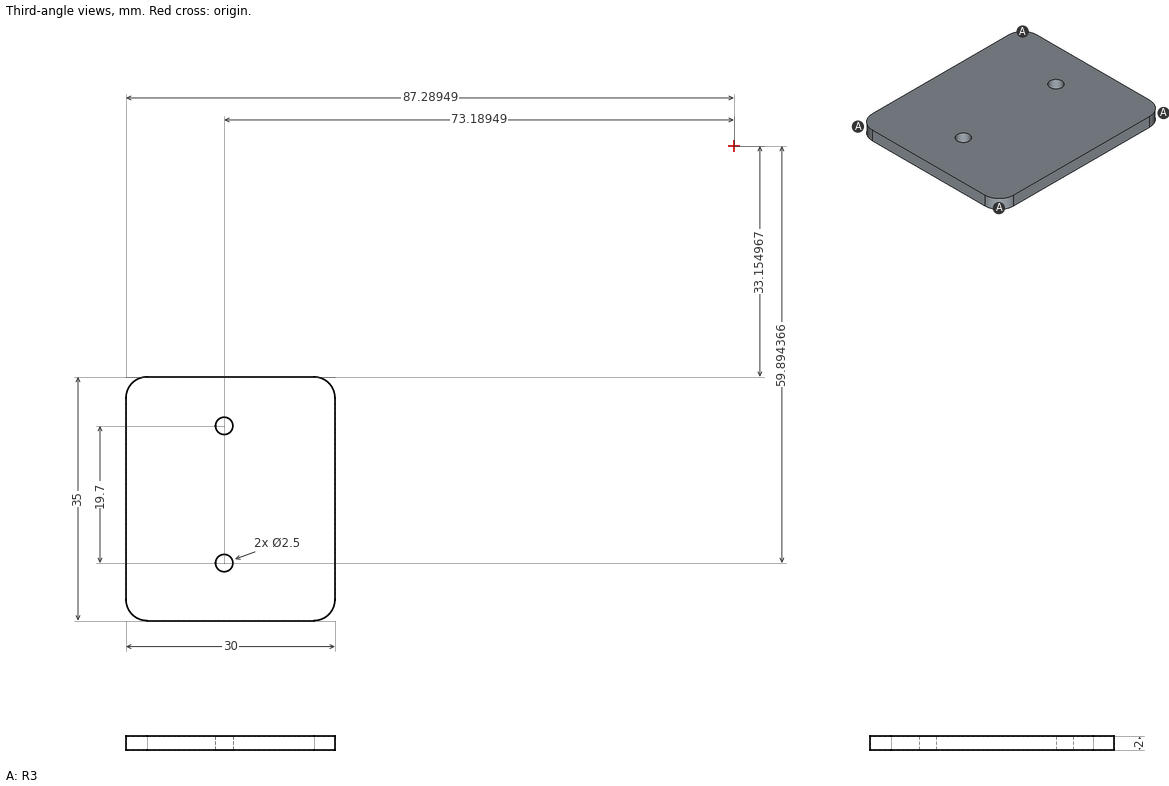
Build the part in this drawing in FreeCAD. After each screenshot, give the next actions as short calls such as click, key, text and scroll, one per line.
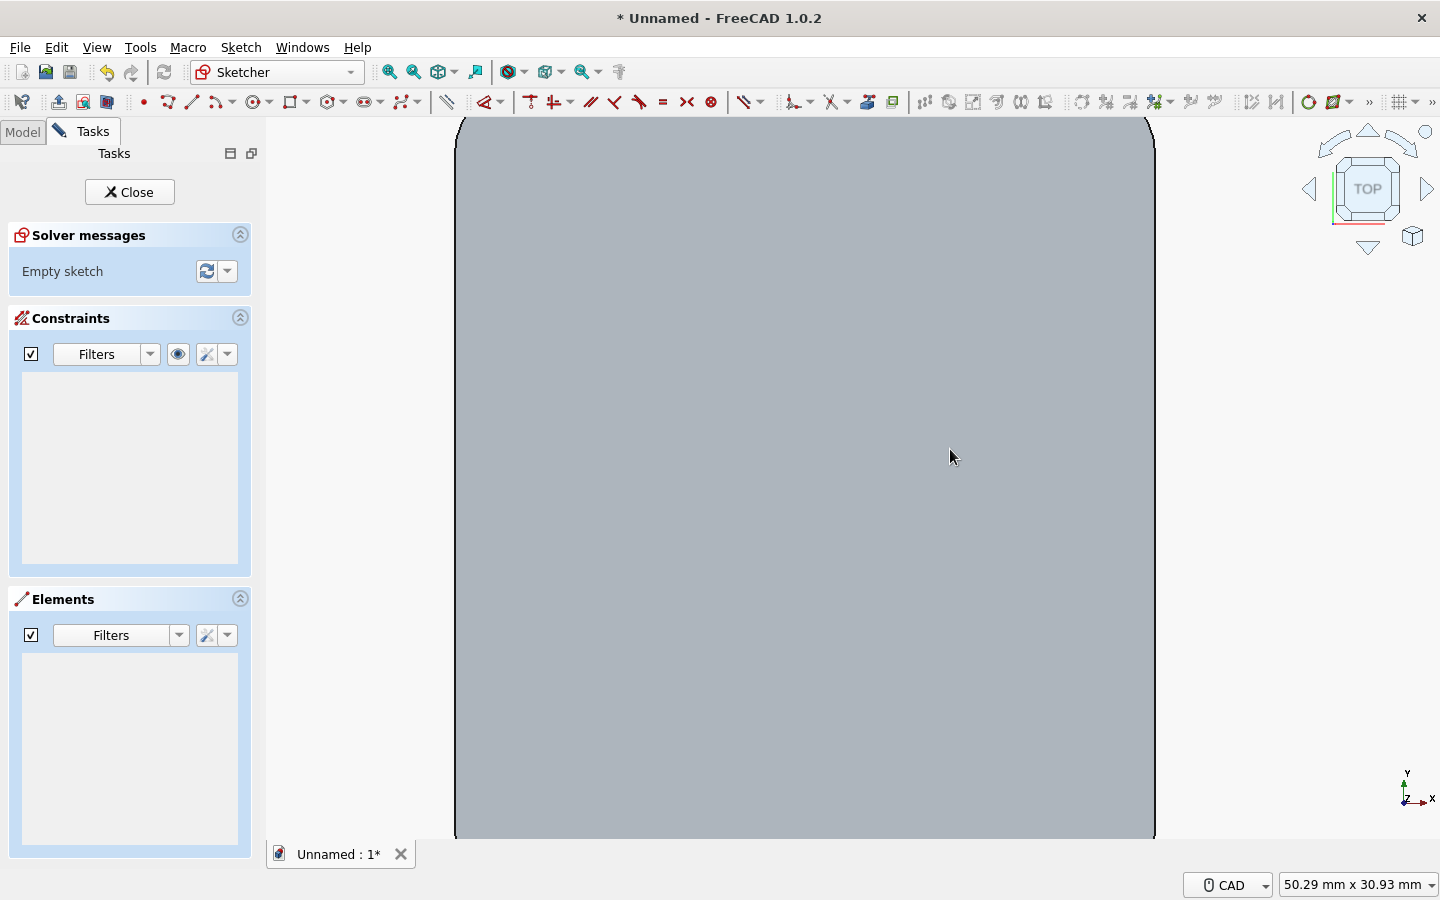
click(254, 102)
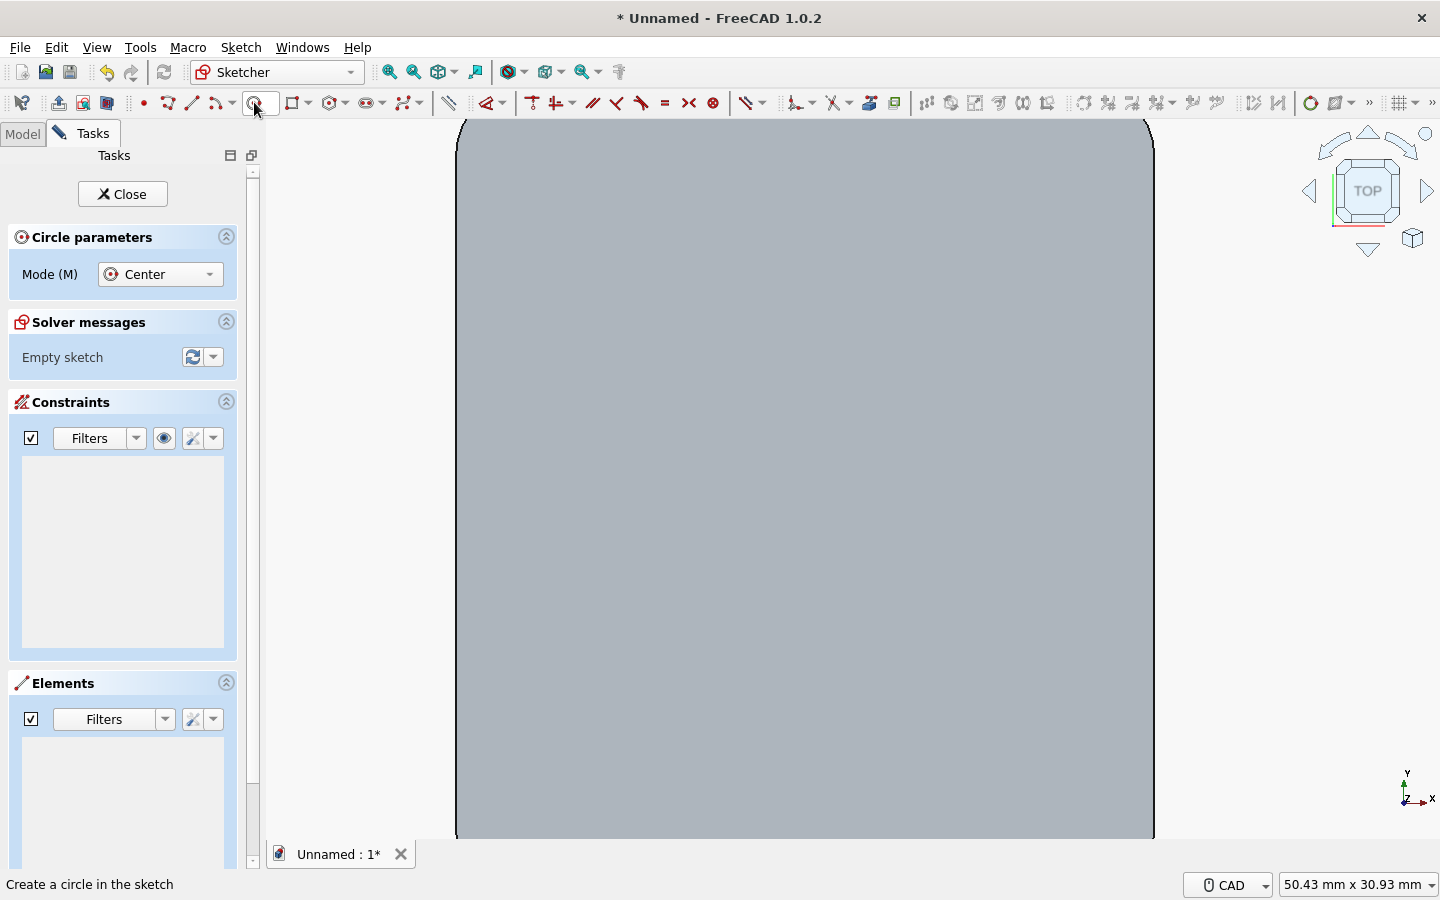
click(784, 708)
move(805, 688)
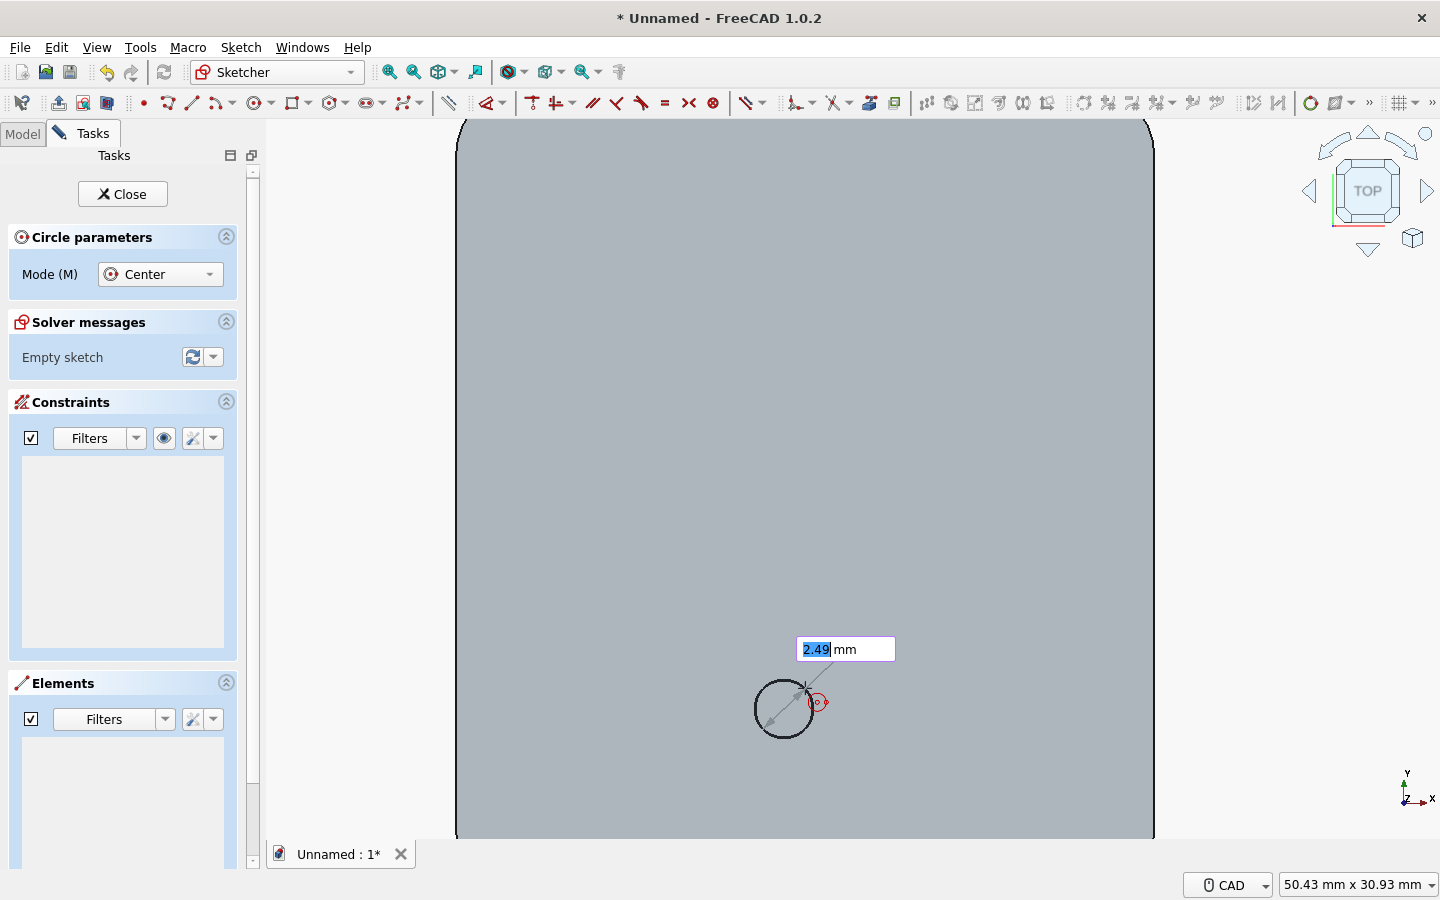
text(2.5)
key(Return)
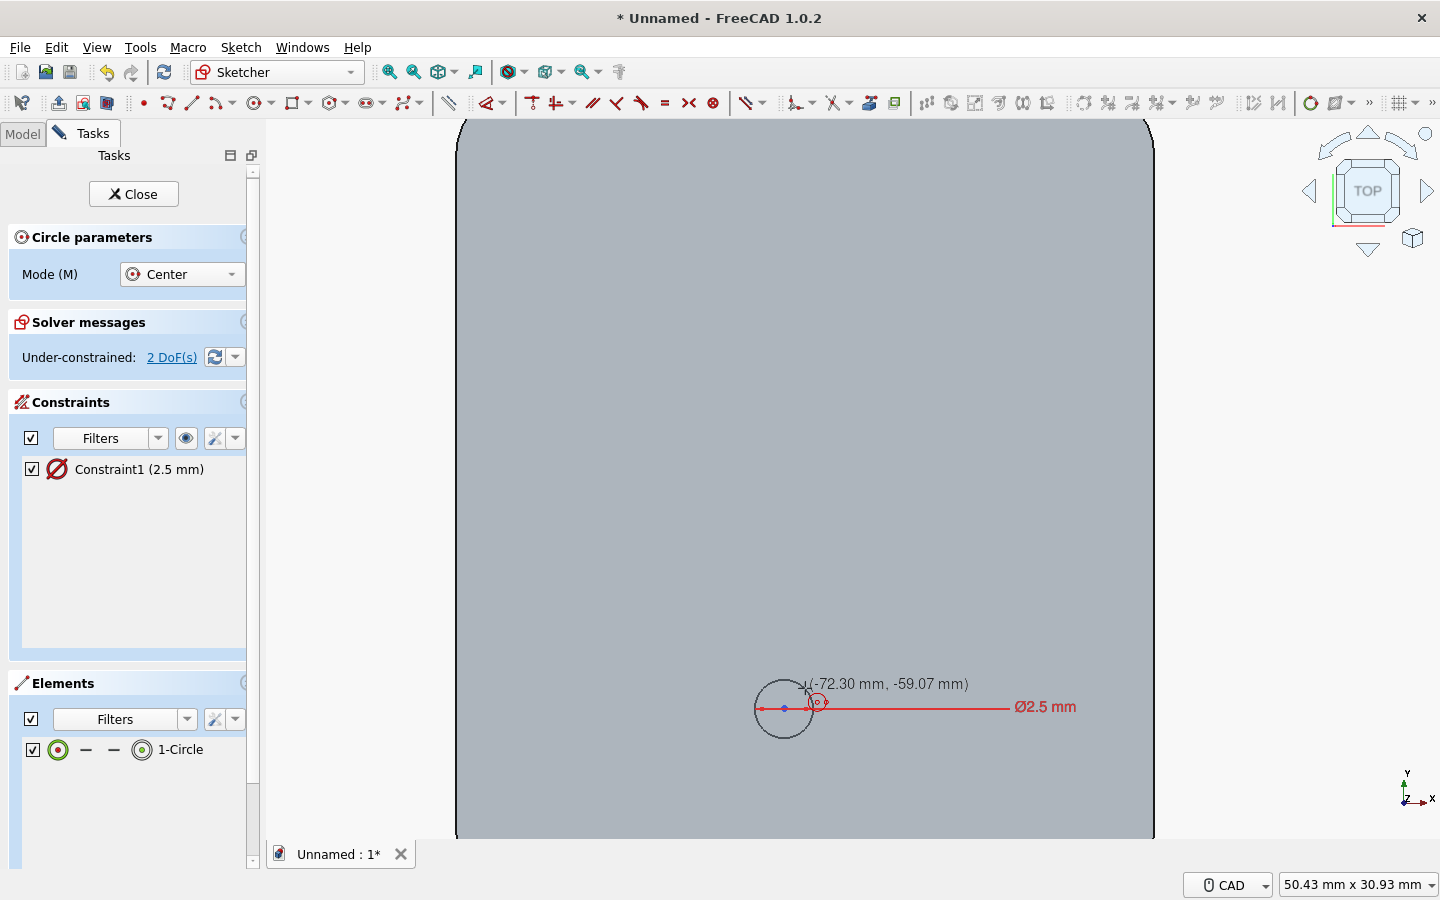
click(784, 249)
move(805, 229)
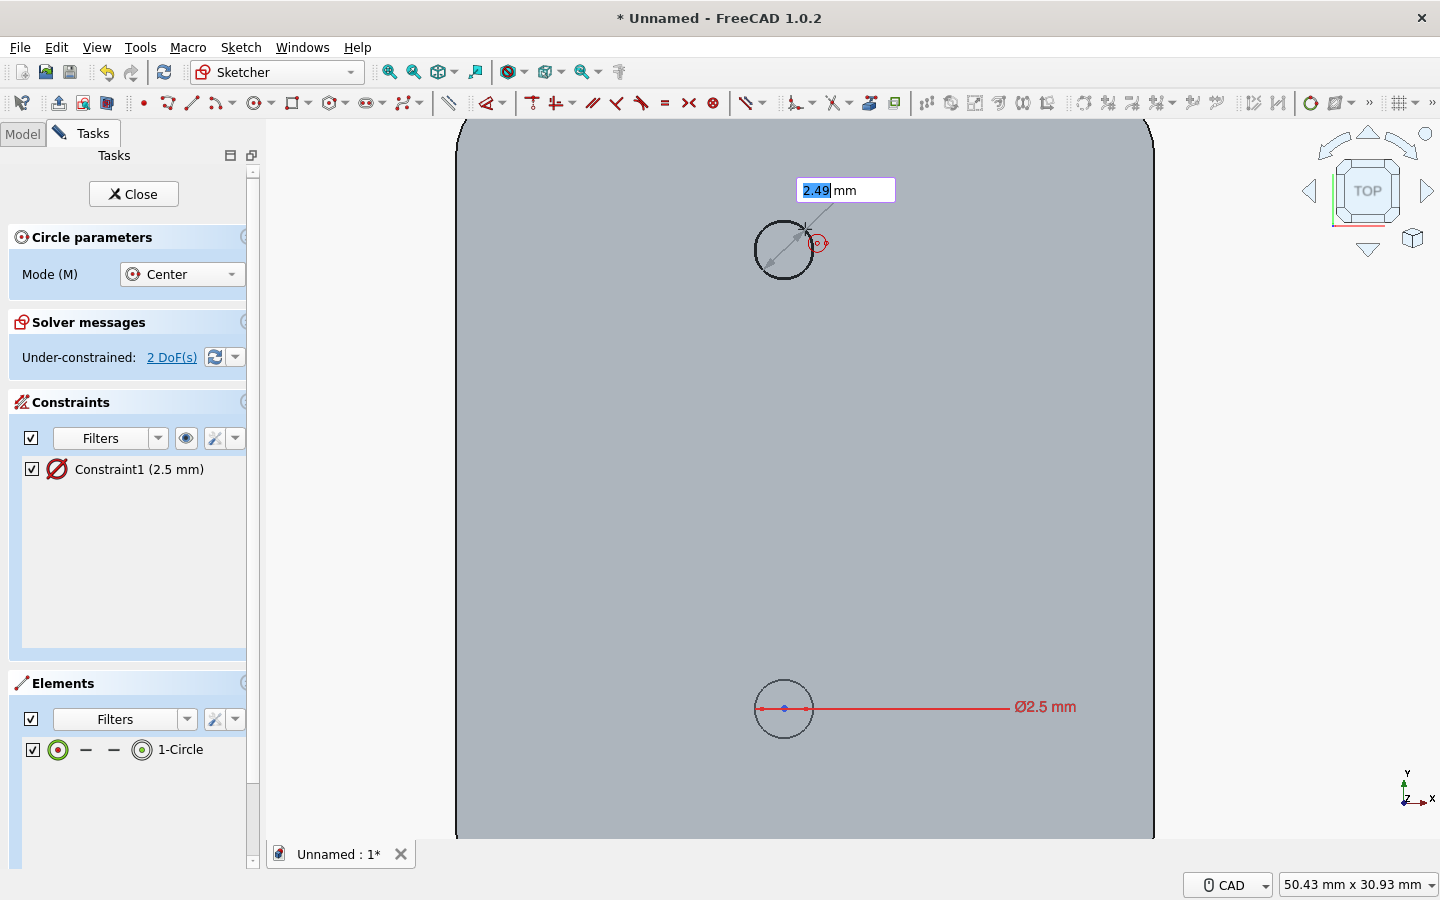
text(2.5)
key(Return)
key(Escape)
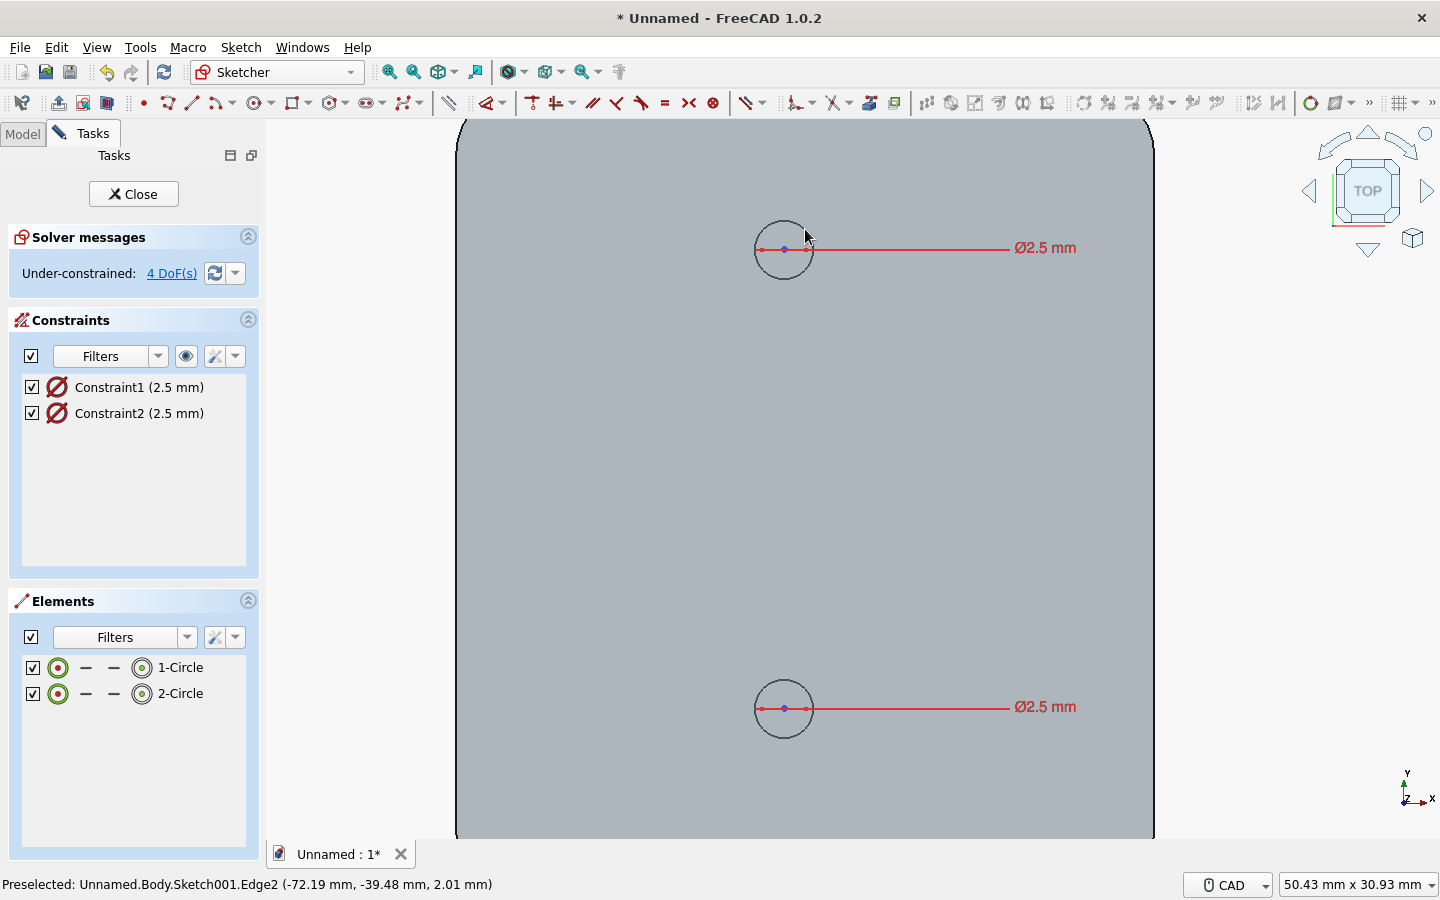
click(784, 709)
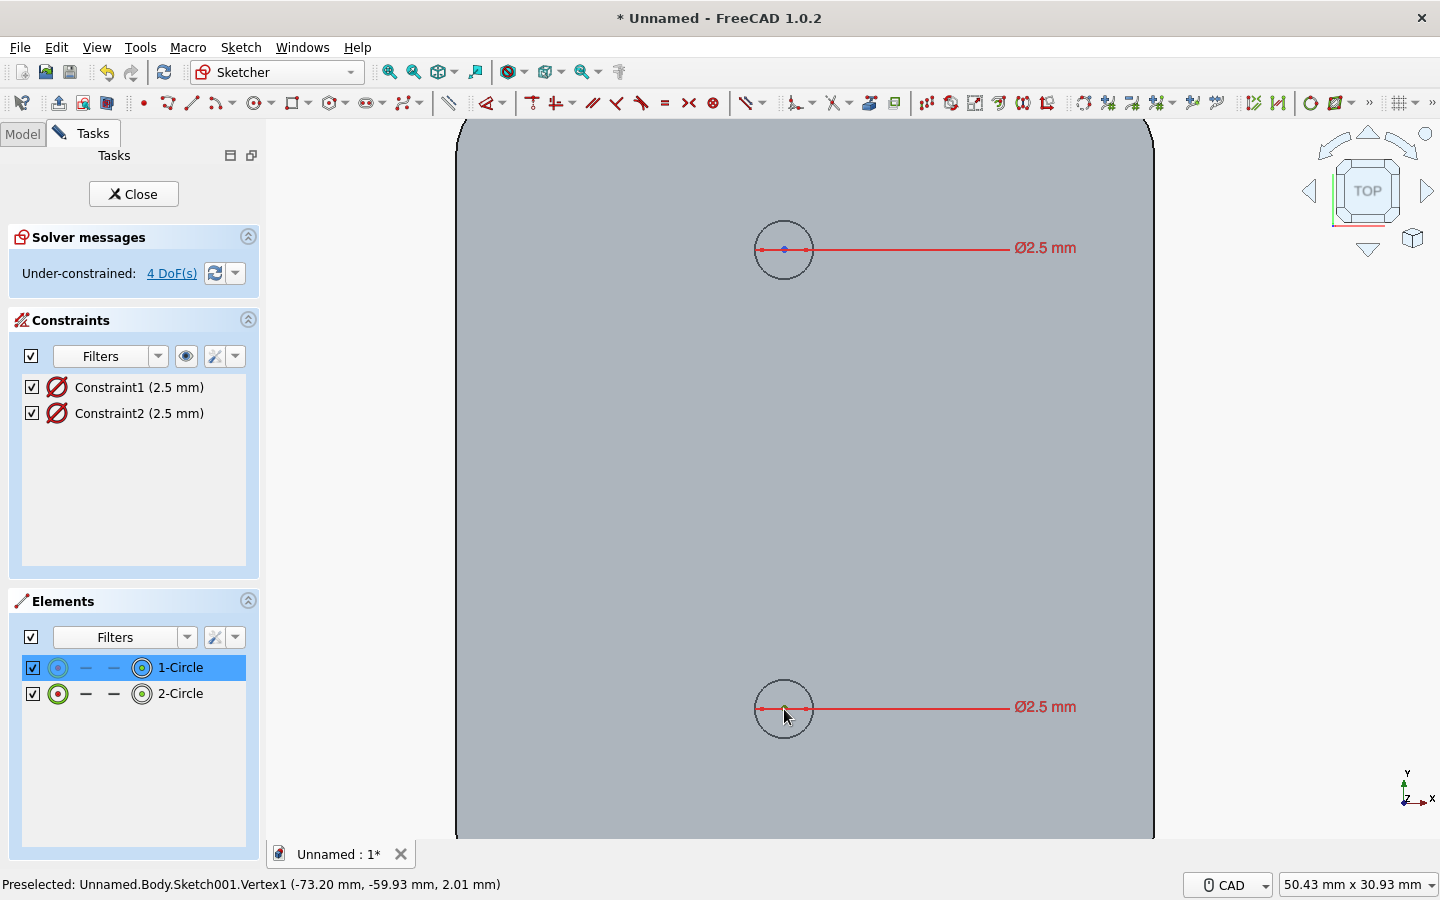
click(784, 250)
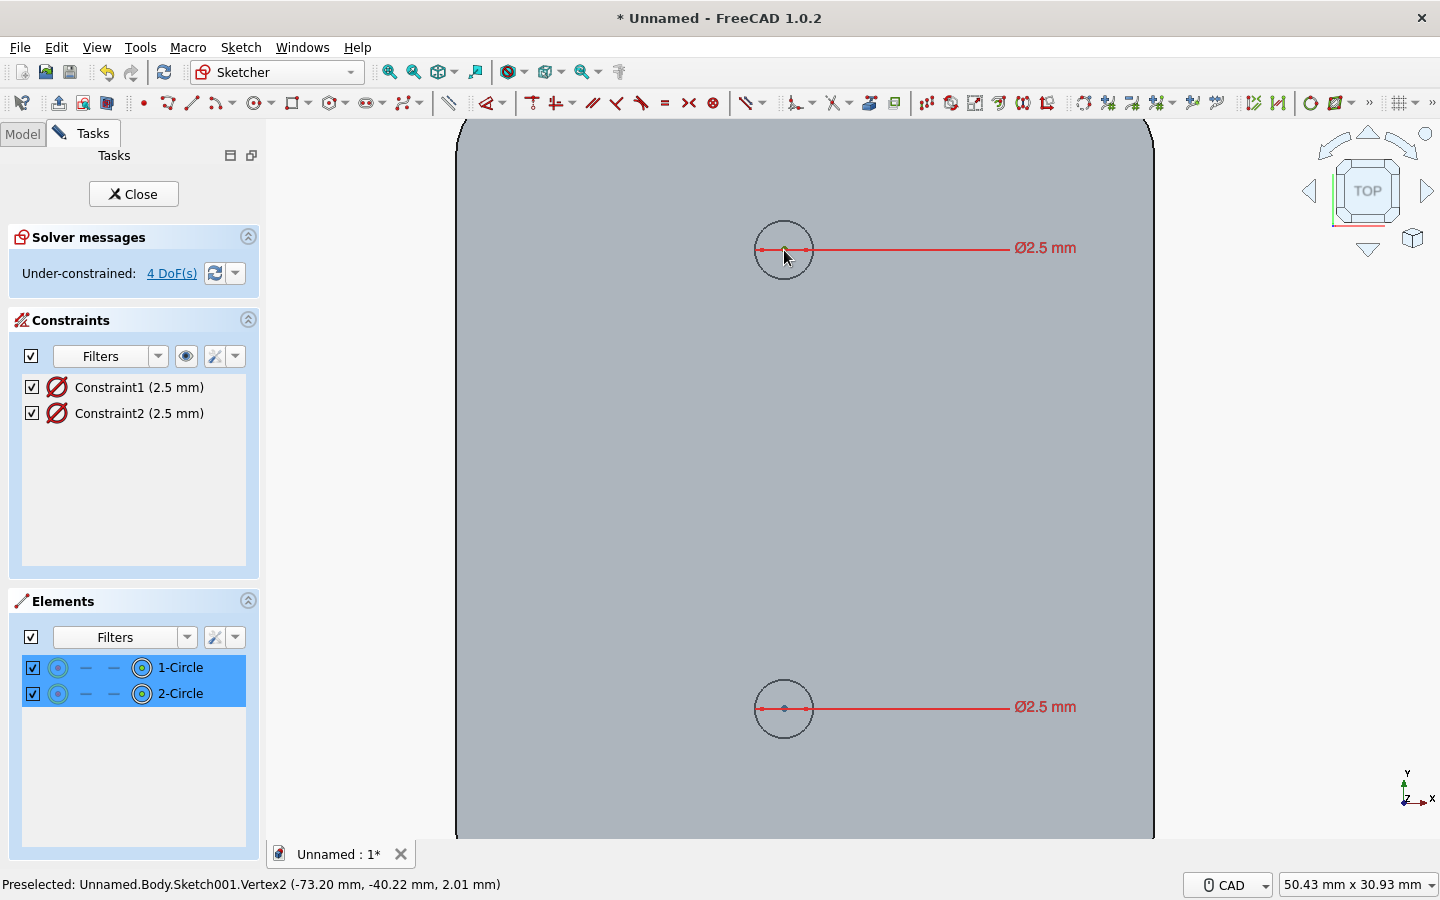
key(v)